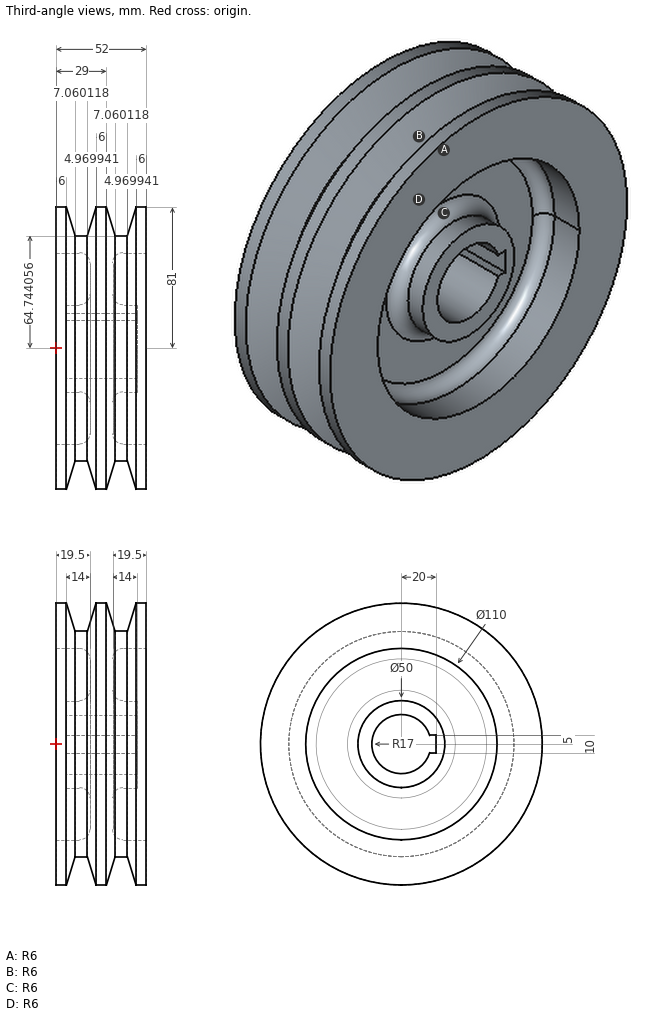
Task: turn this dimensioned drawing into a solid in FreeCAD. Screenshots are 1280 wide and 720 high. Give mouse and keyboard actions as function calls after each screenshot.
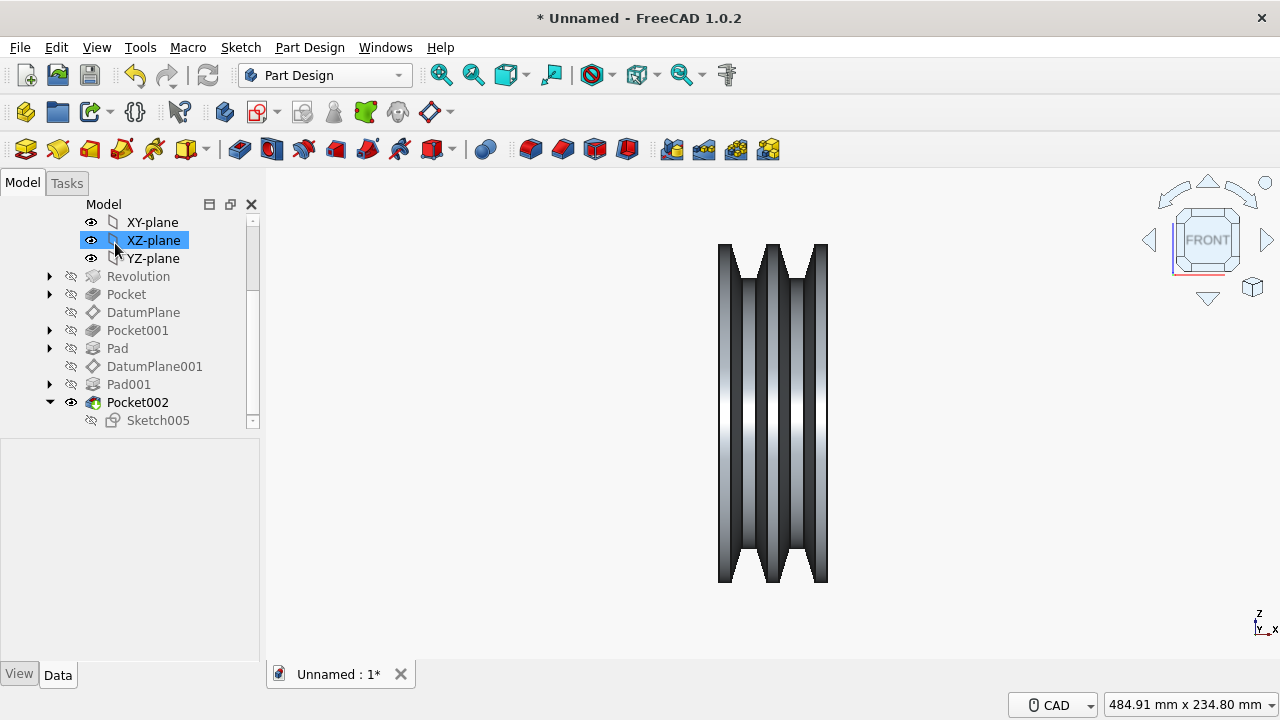
key(3)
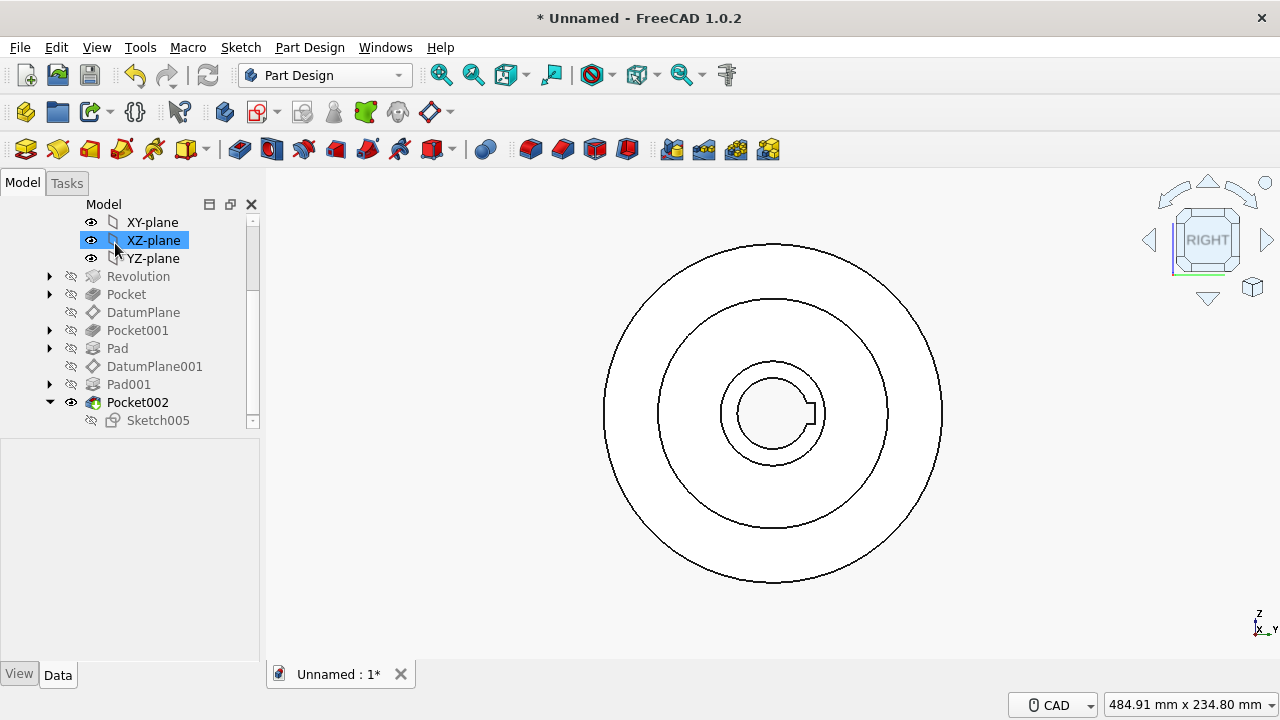
key(5)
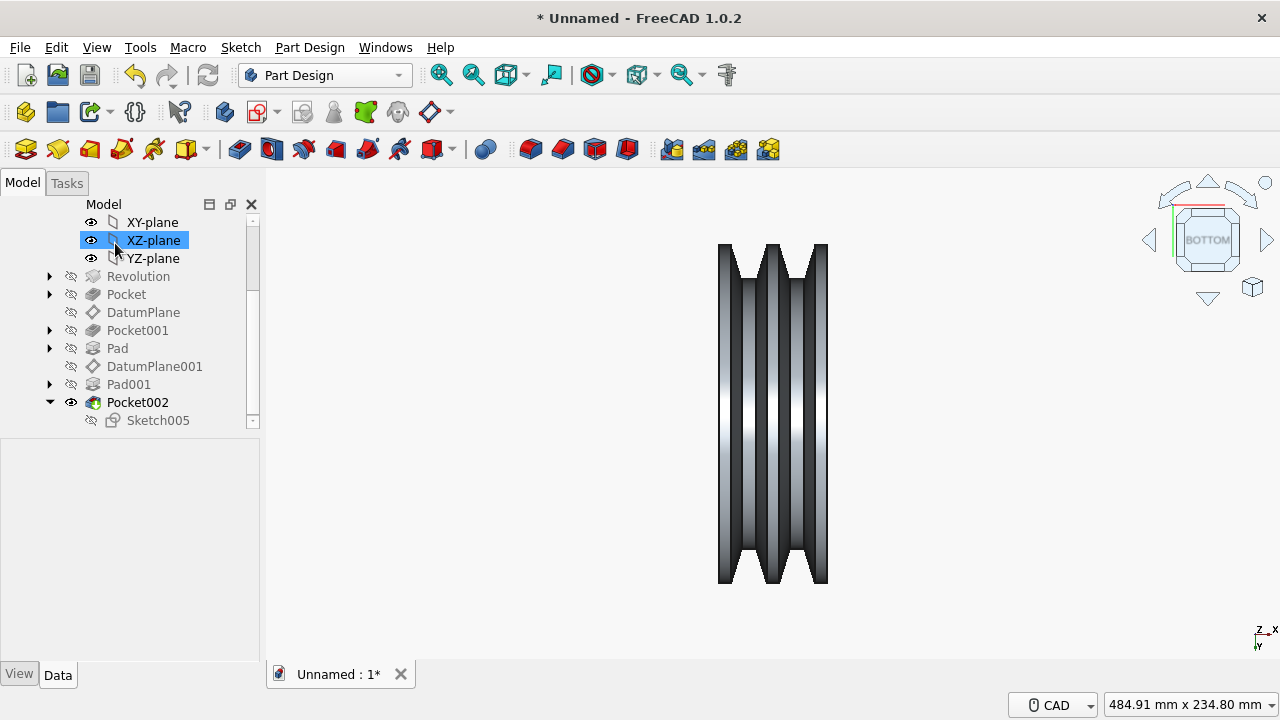
key(4)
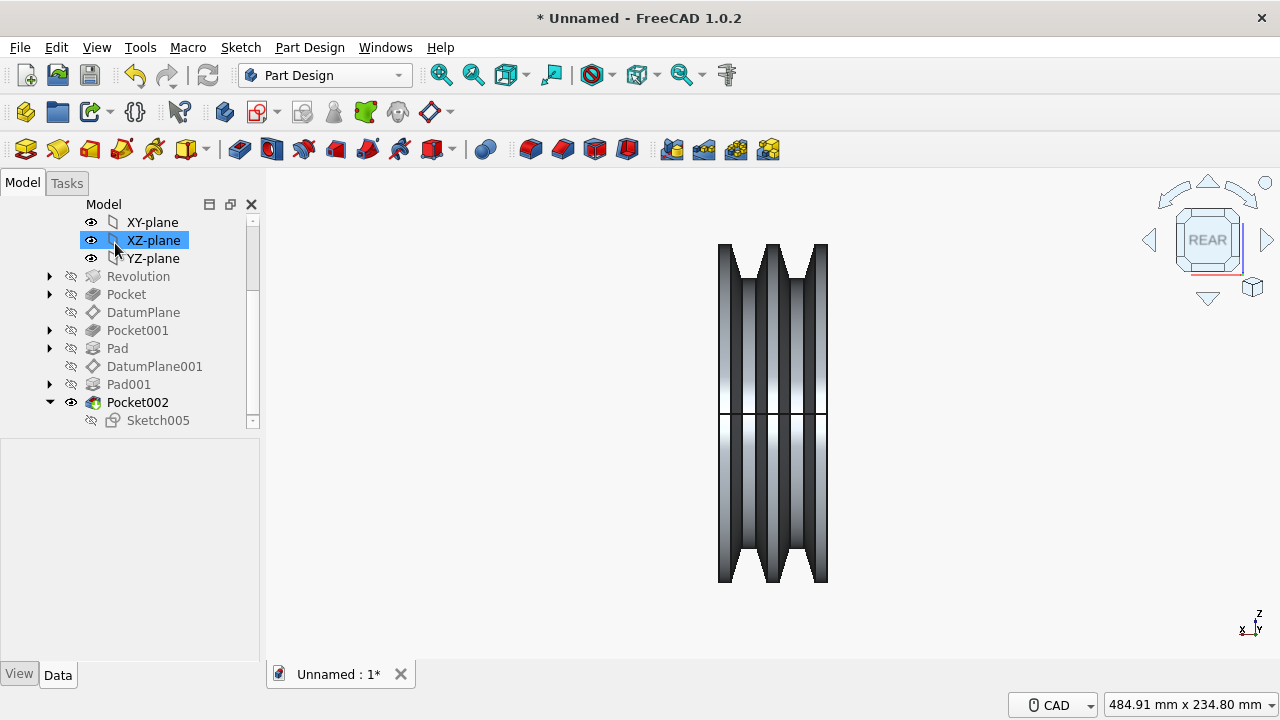
key(6)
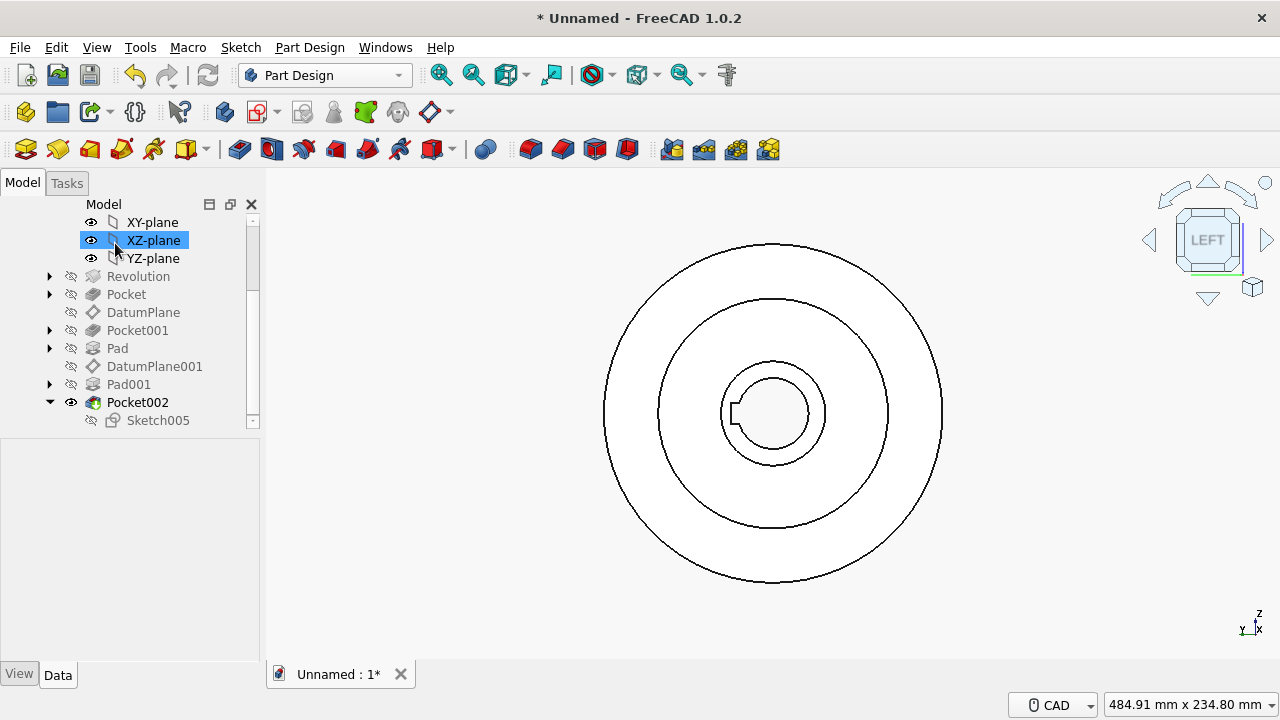
key(v)
key(3)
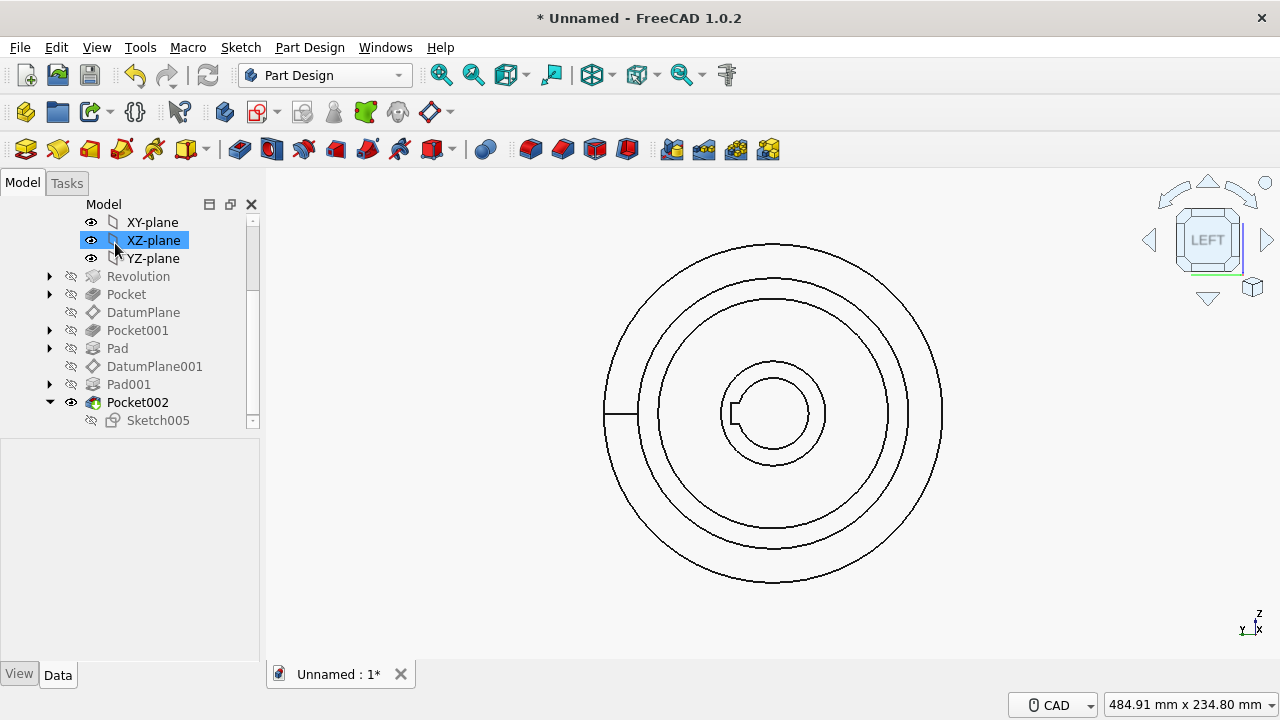
key(0)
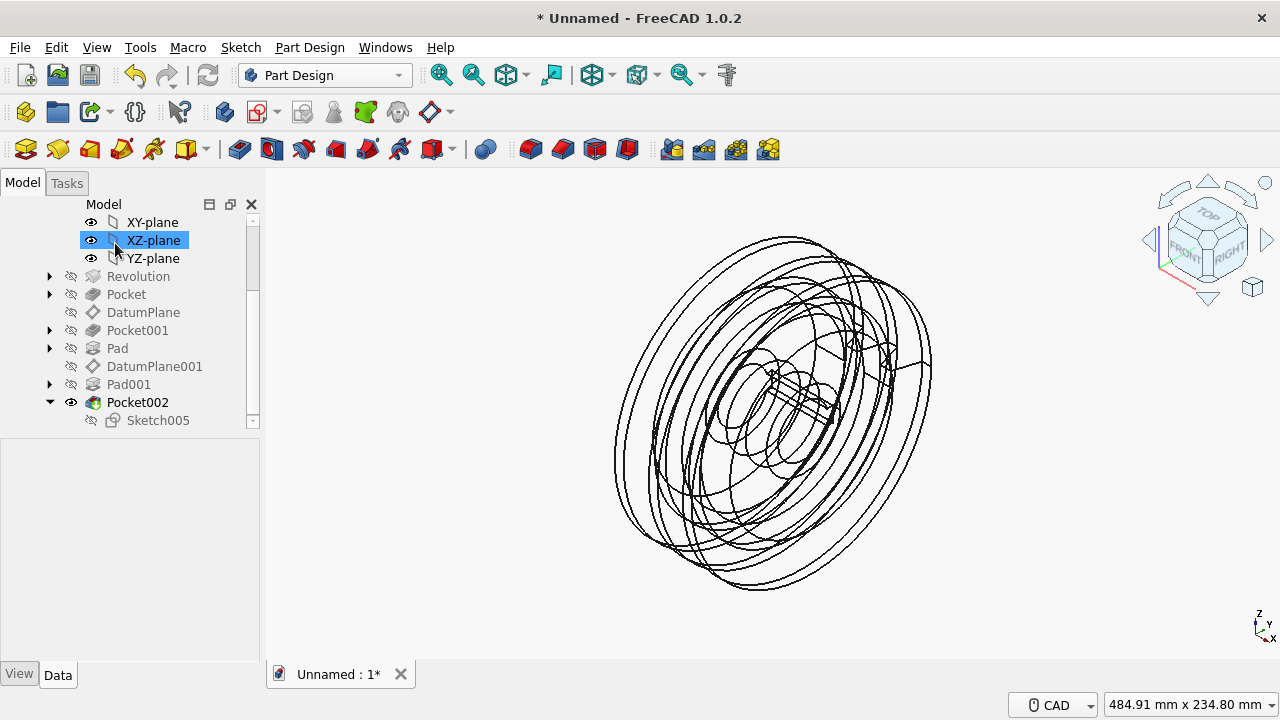
click(717, 511)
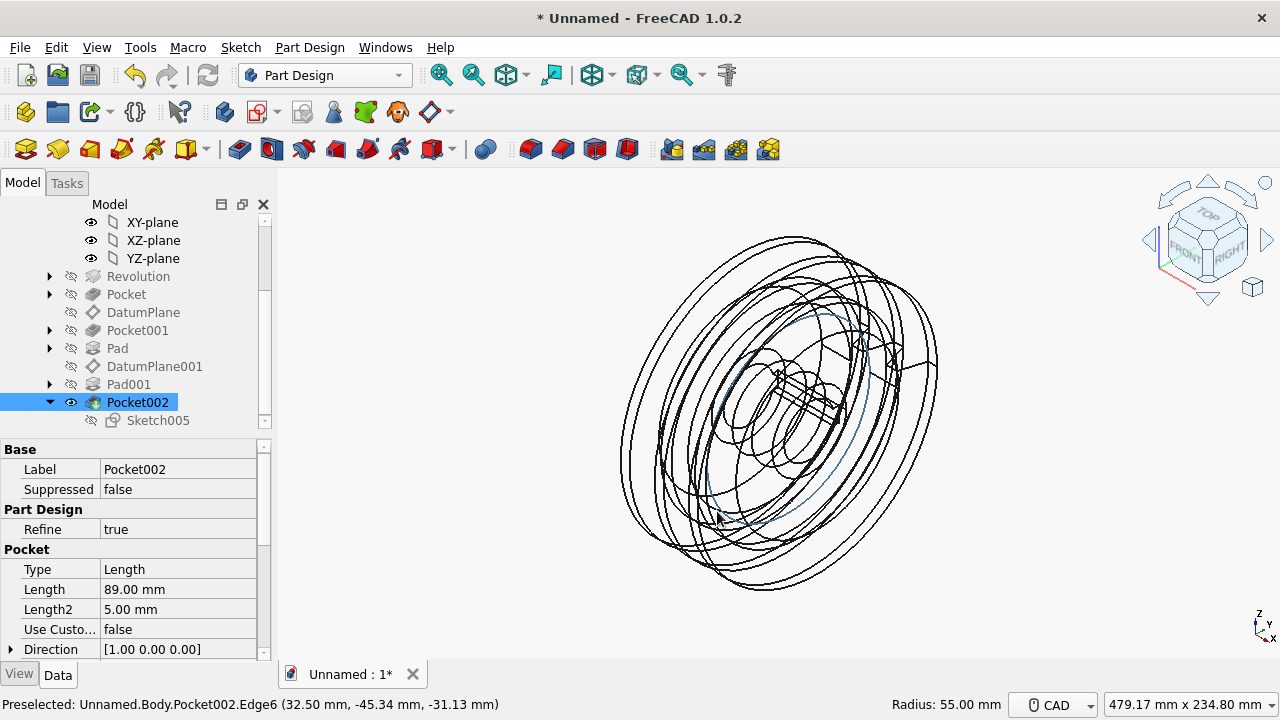
key(v)
key(1)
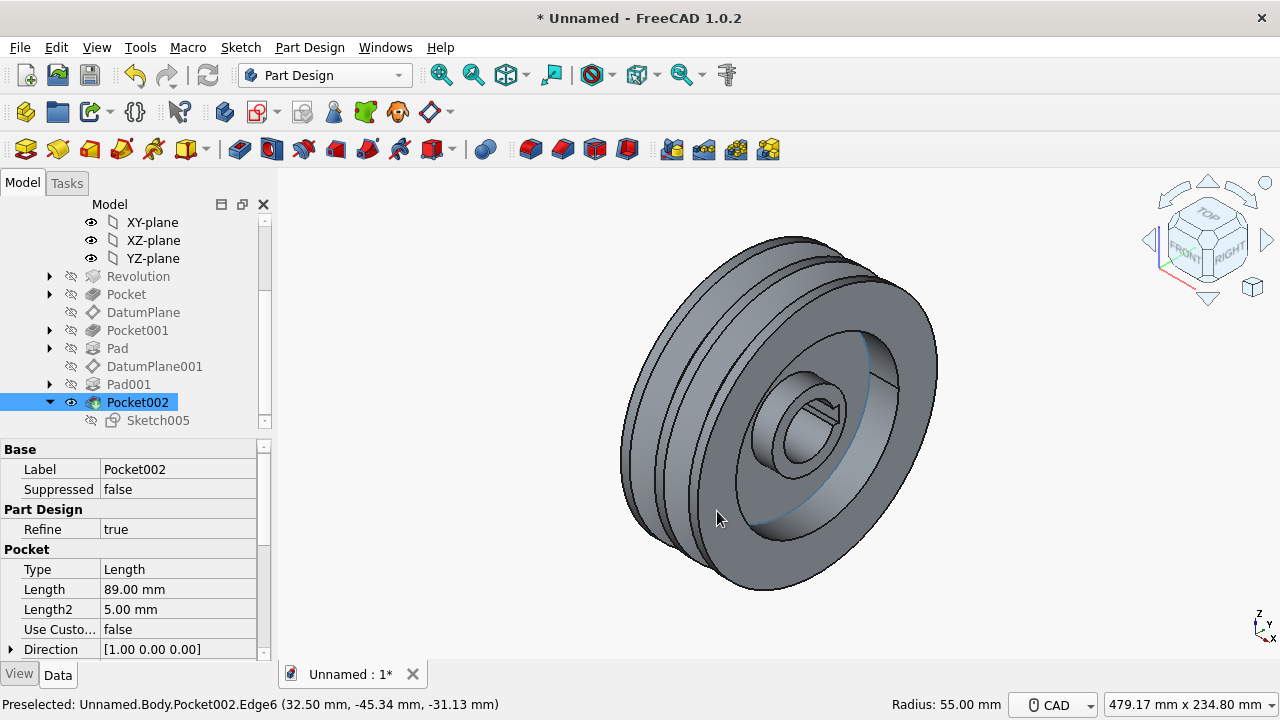
click(532, 150)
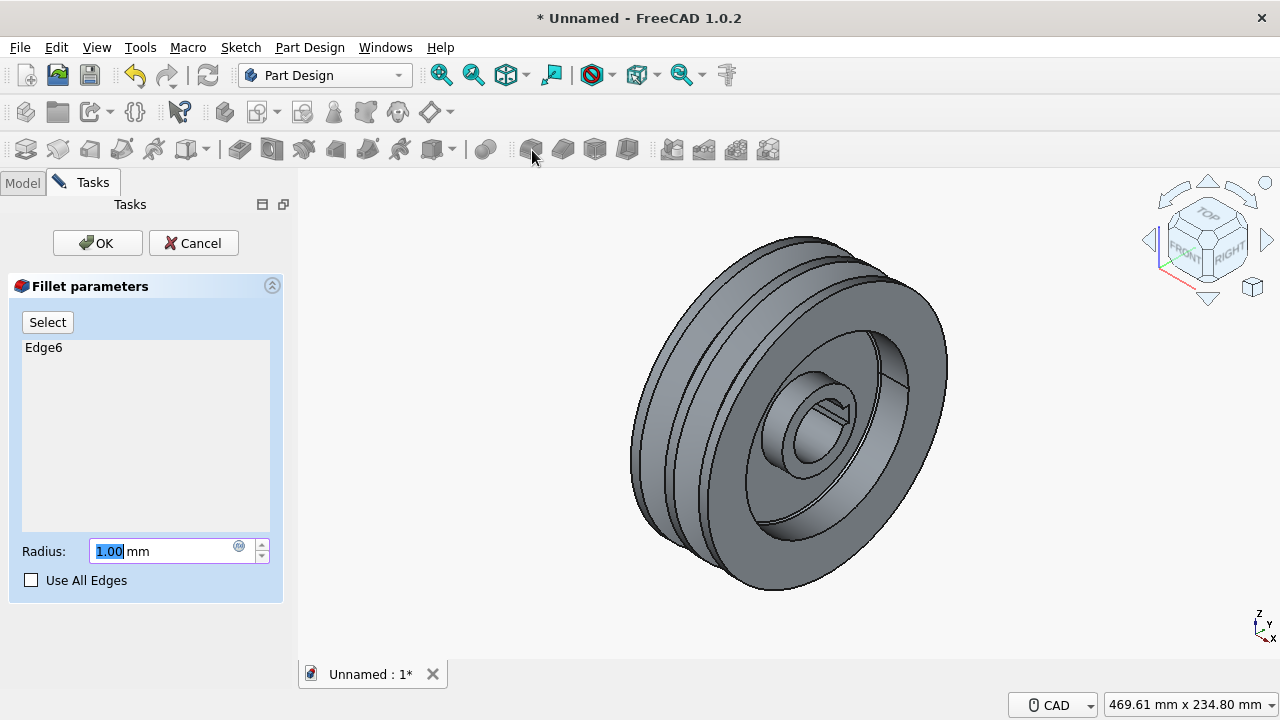
text(6)
key(Tab)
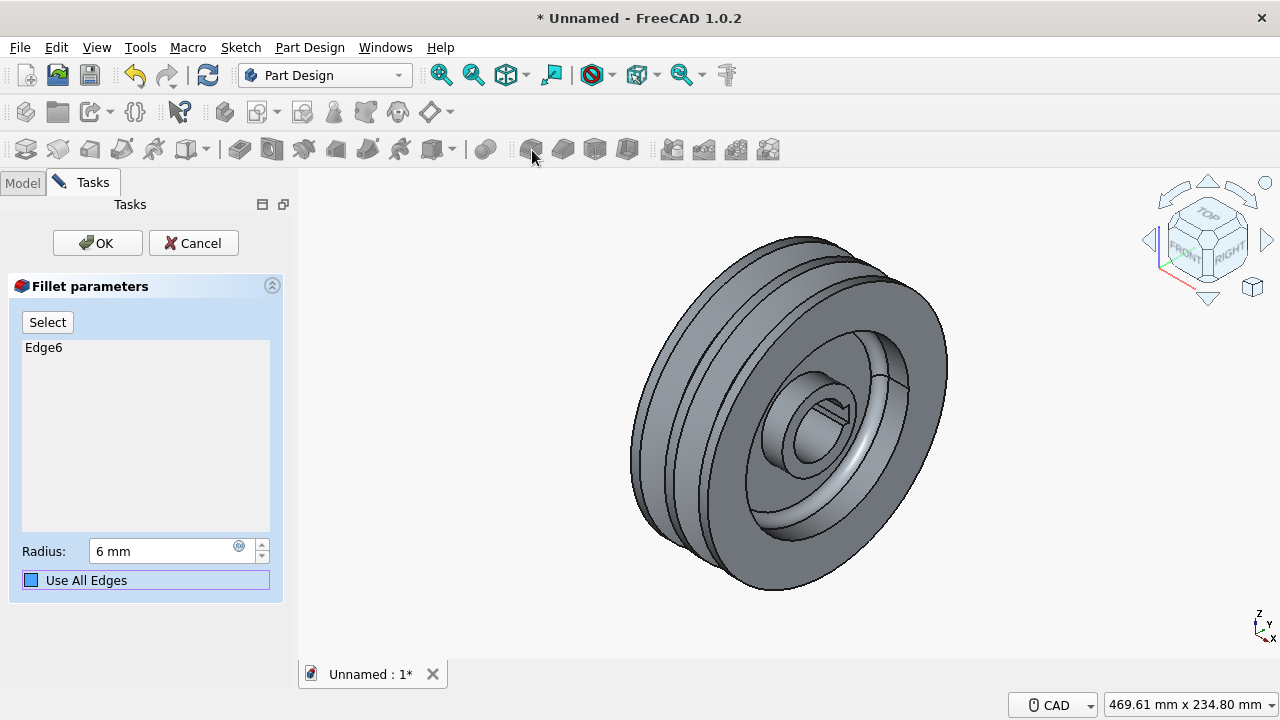
click(98, 243)